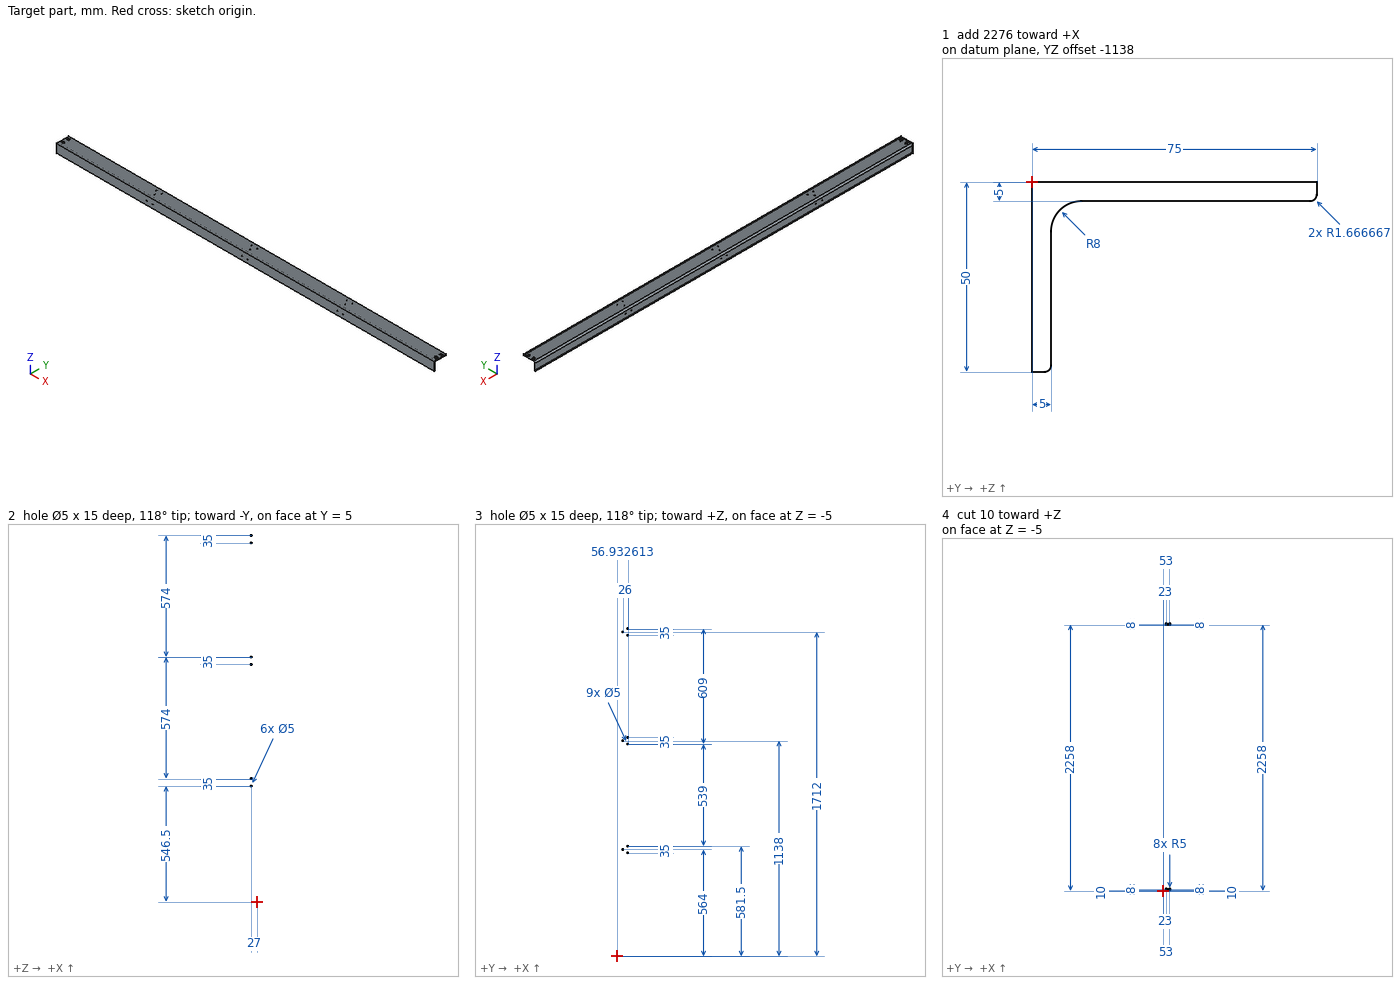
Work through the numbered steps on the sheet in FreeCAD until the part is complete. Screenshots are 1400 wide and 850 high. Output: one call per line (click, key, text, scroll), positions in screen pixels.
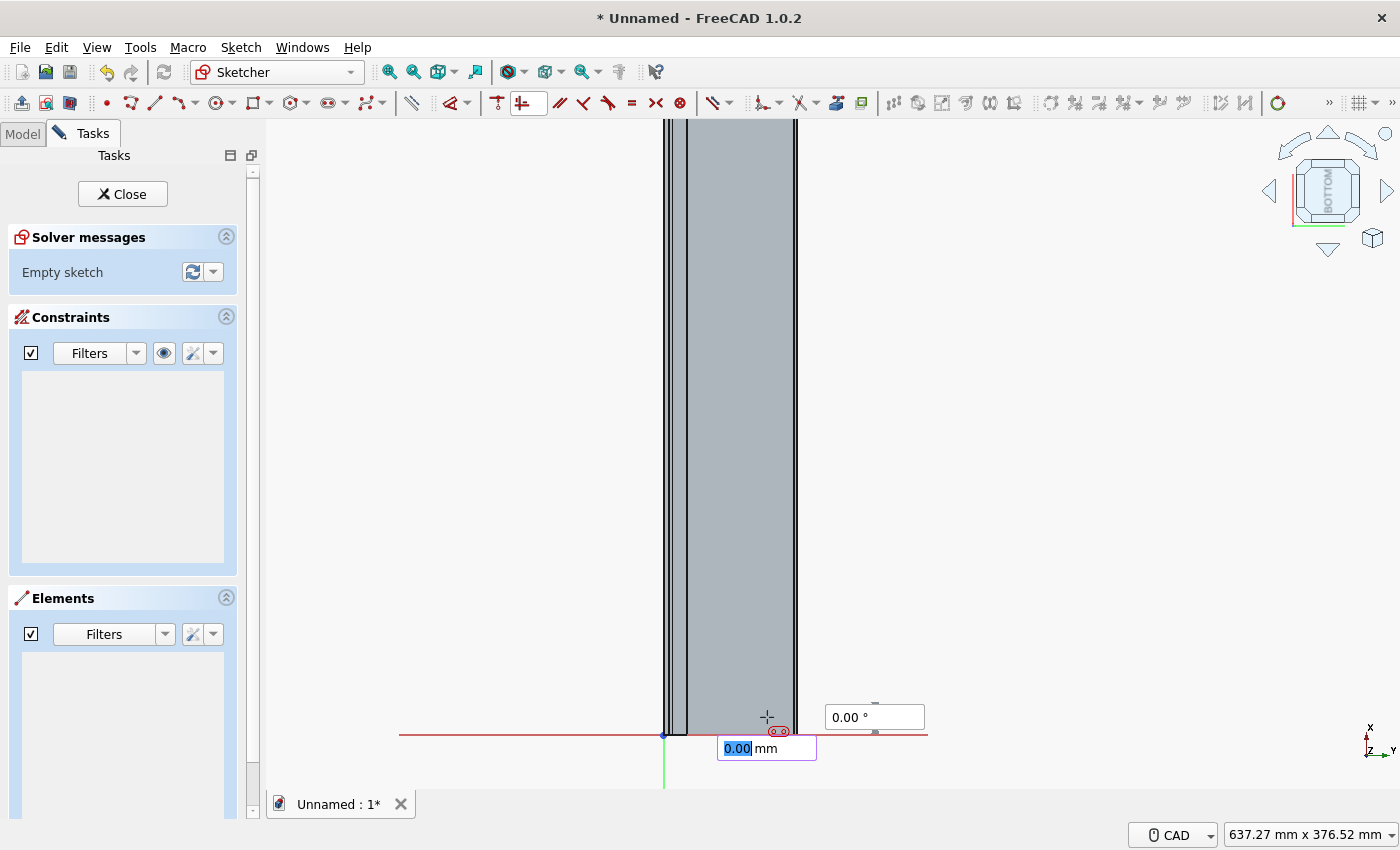
click(767, 703)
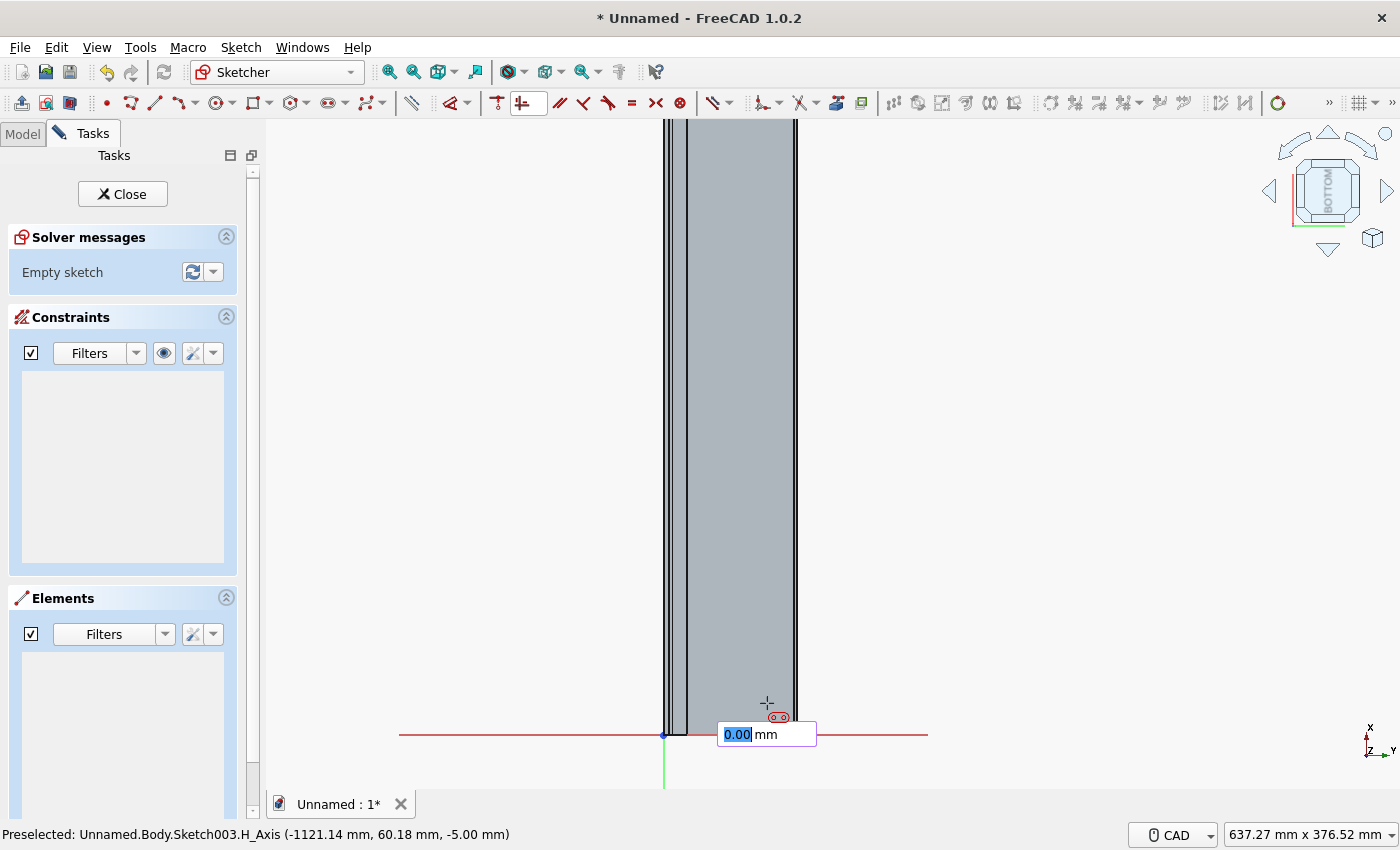
scroll(758, 710, up, 3)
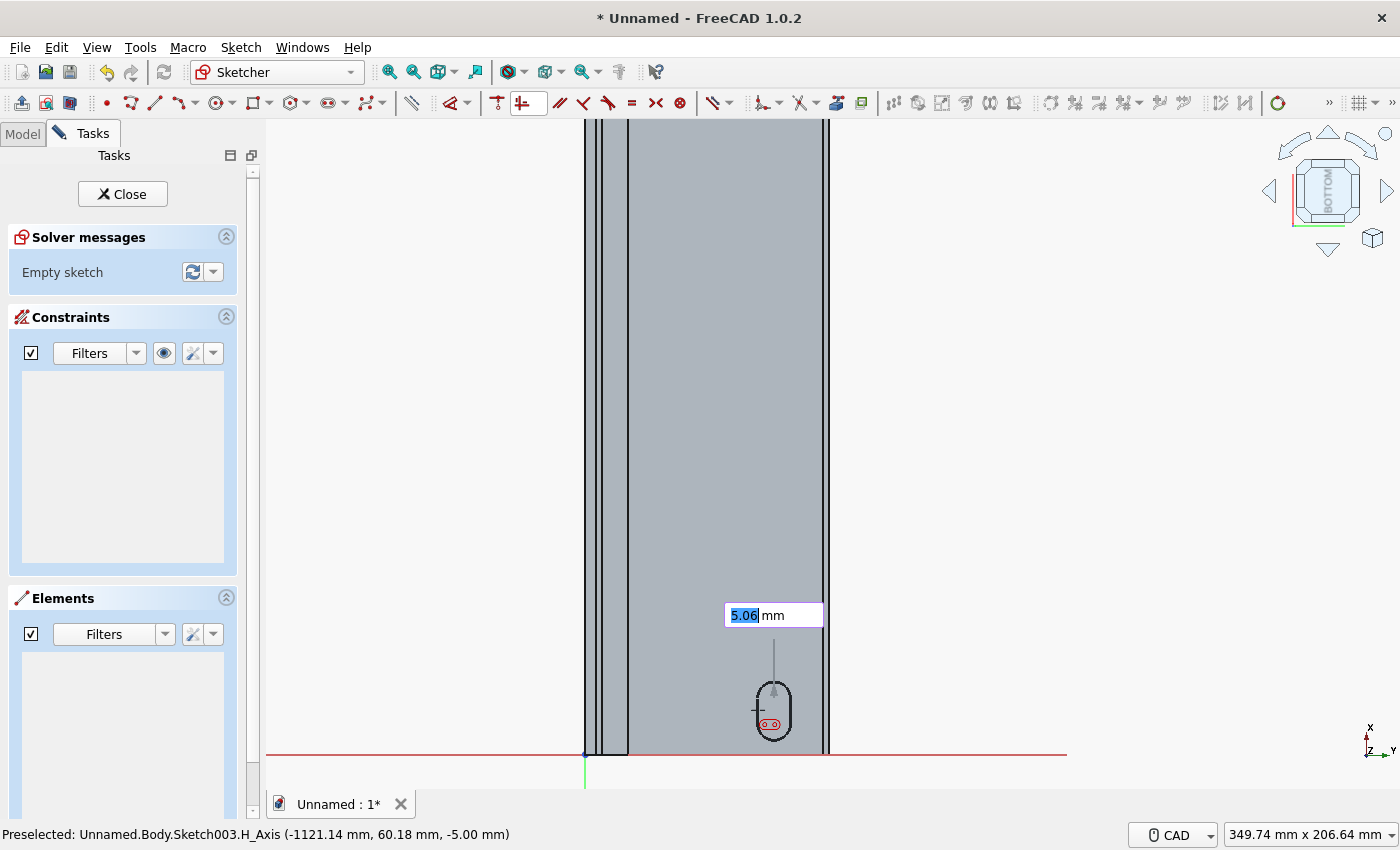
click(757, 709)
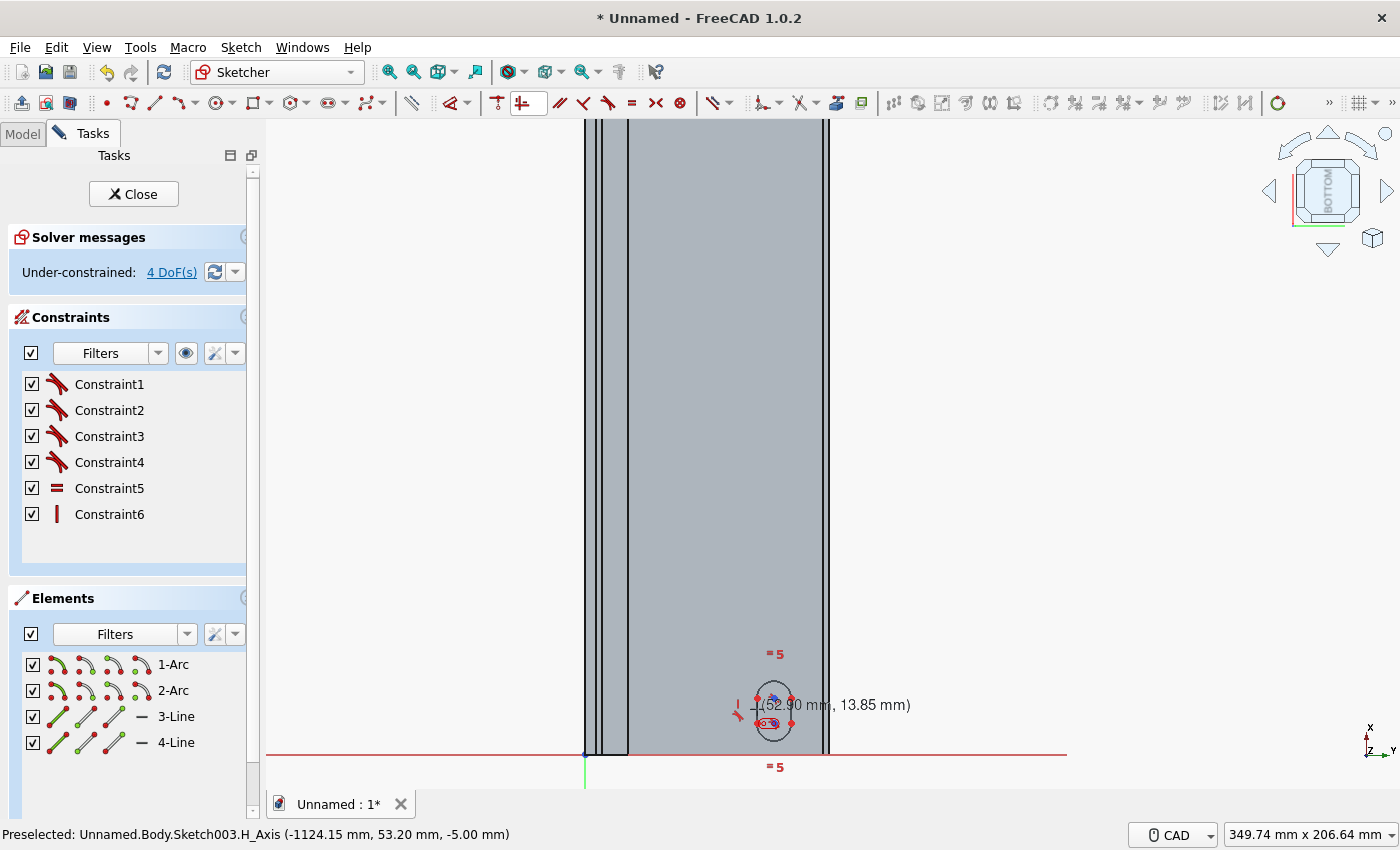
scroll(676, 722, up, 2)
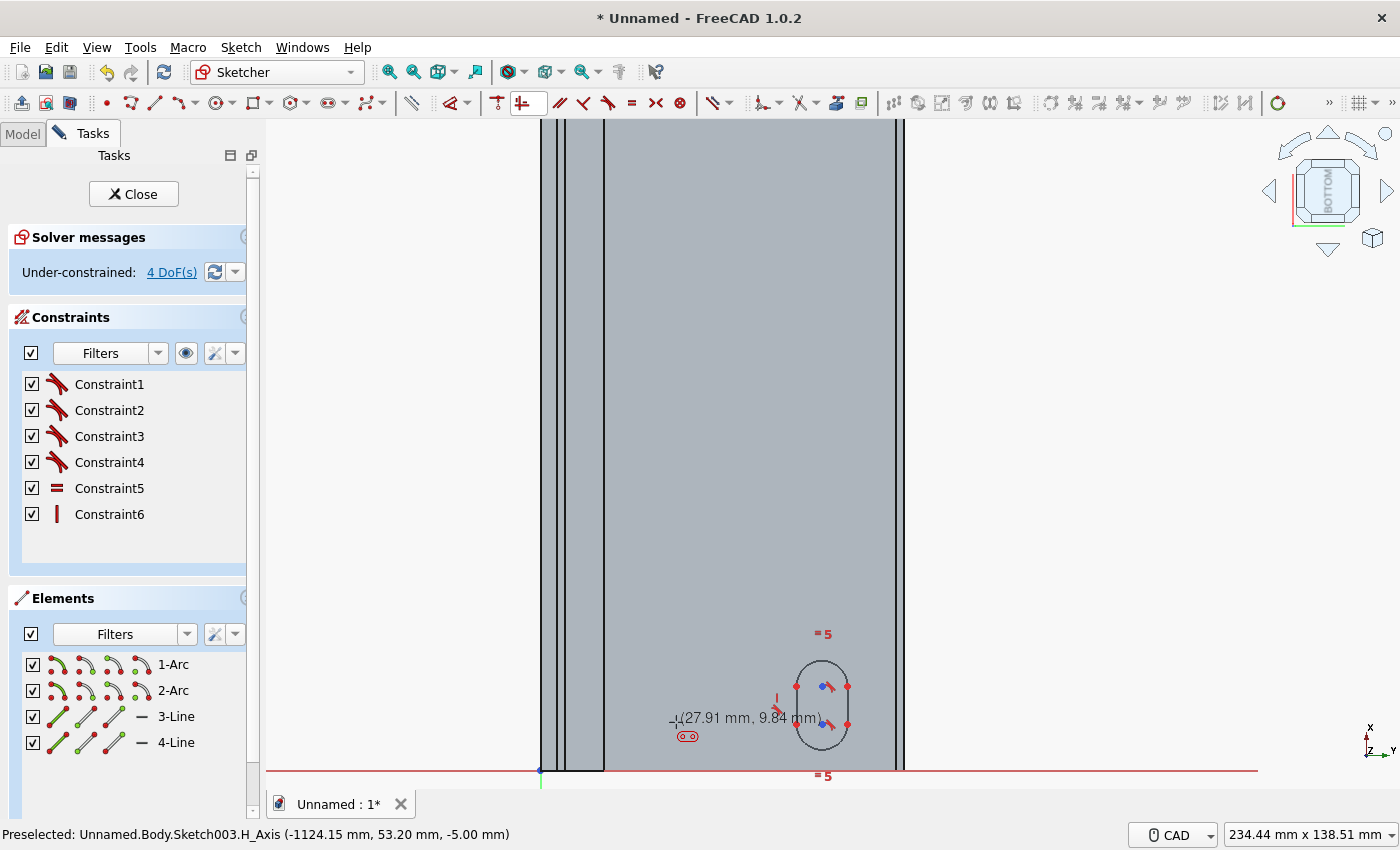
scroll(768, 725, down, 15)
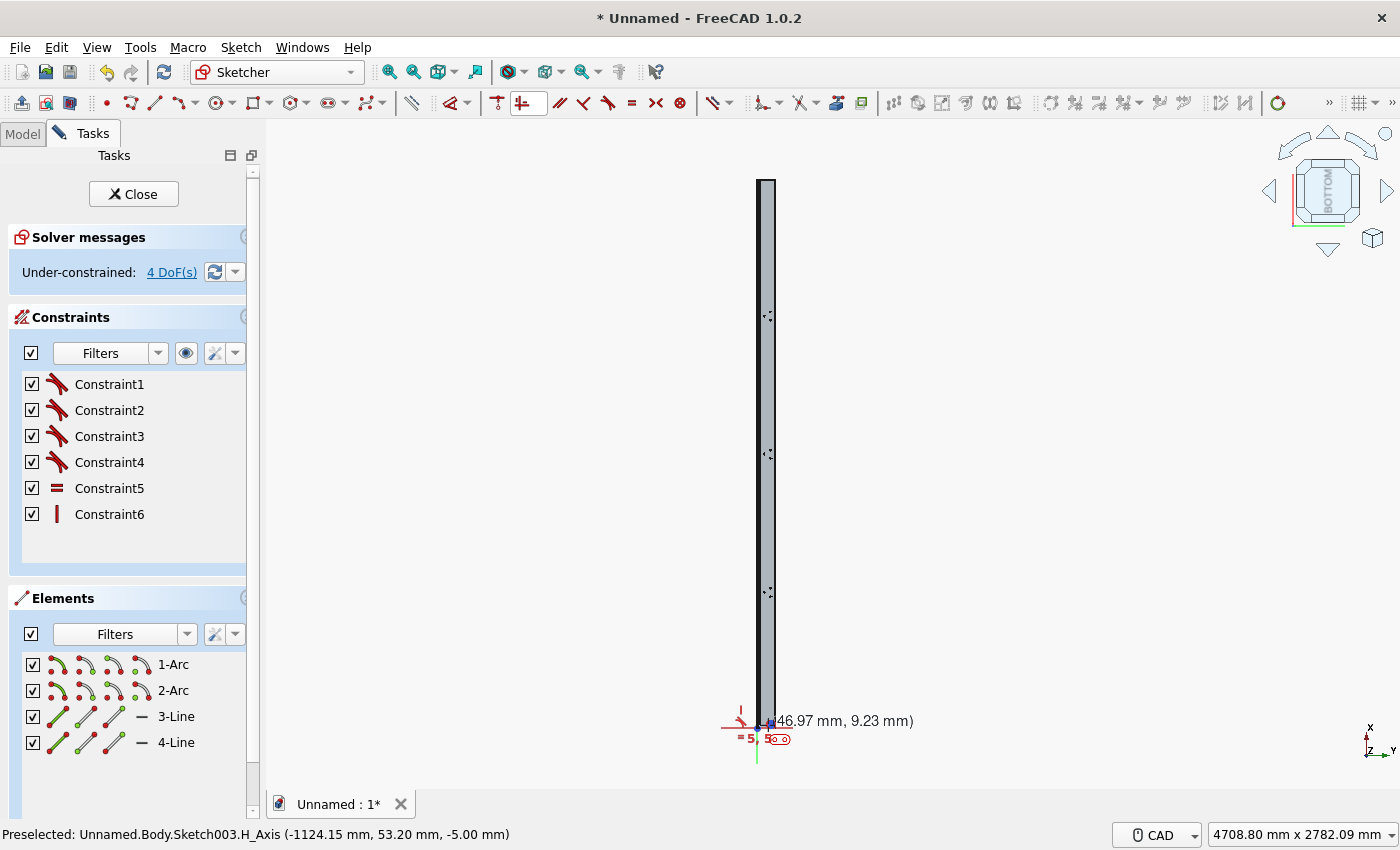
scroll(764, 726, up, 10)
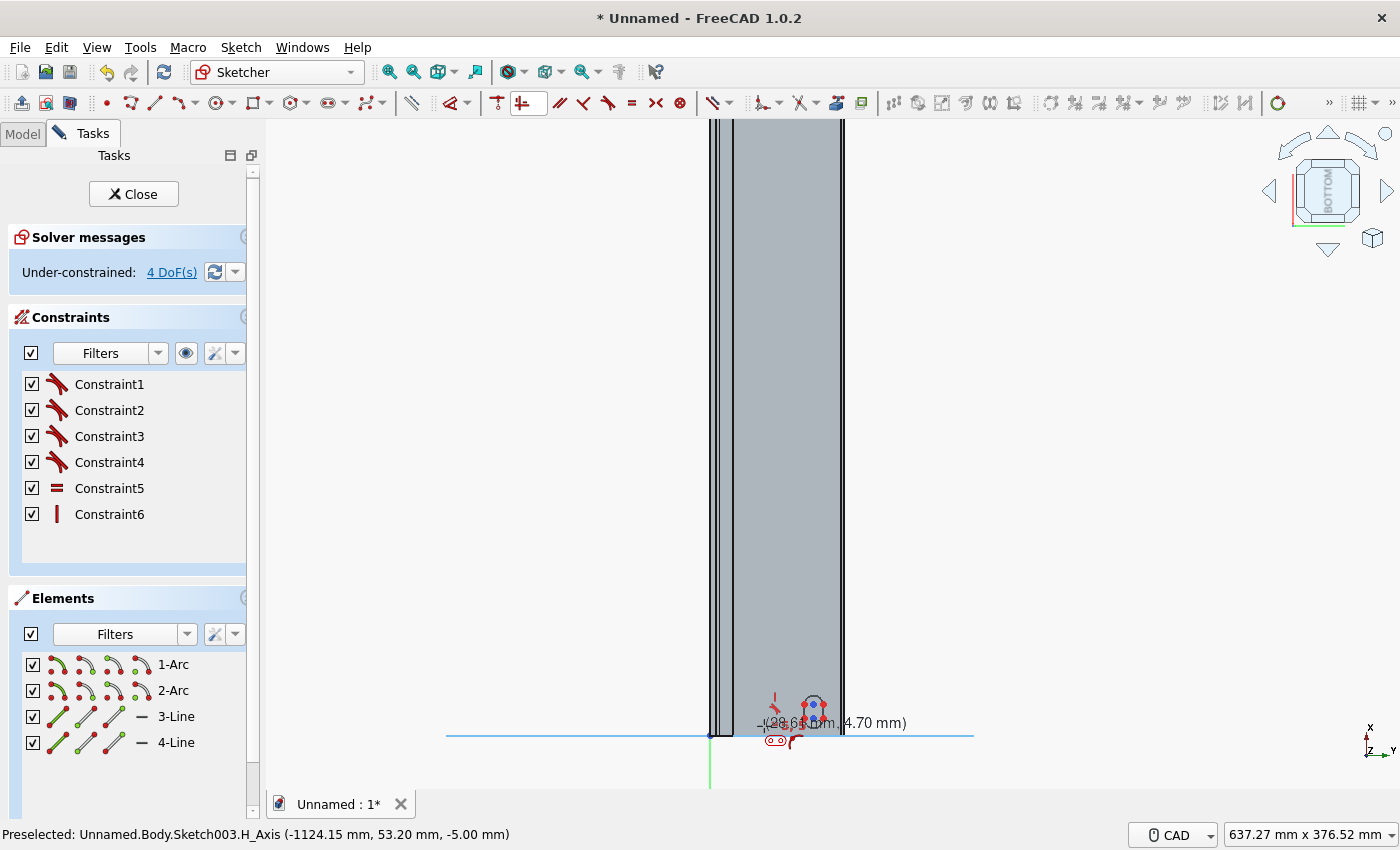
click(760, 718)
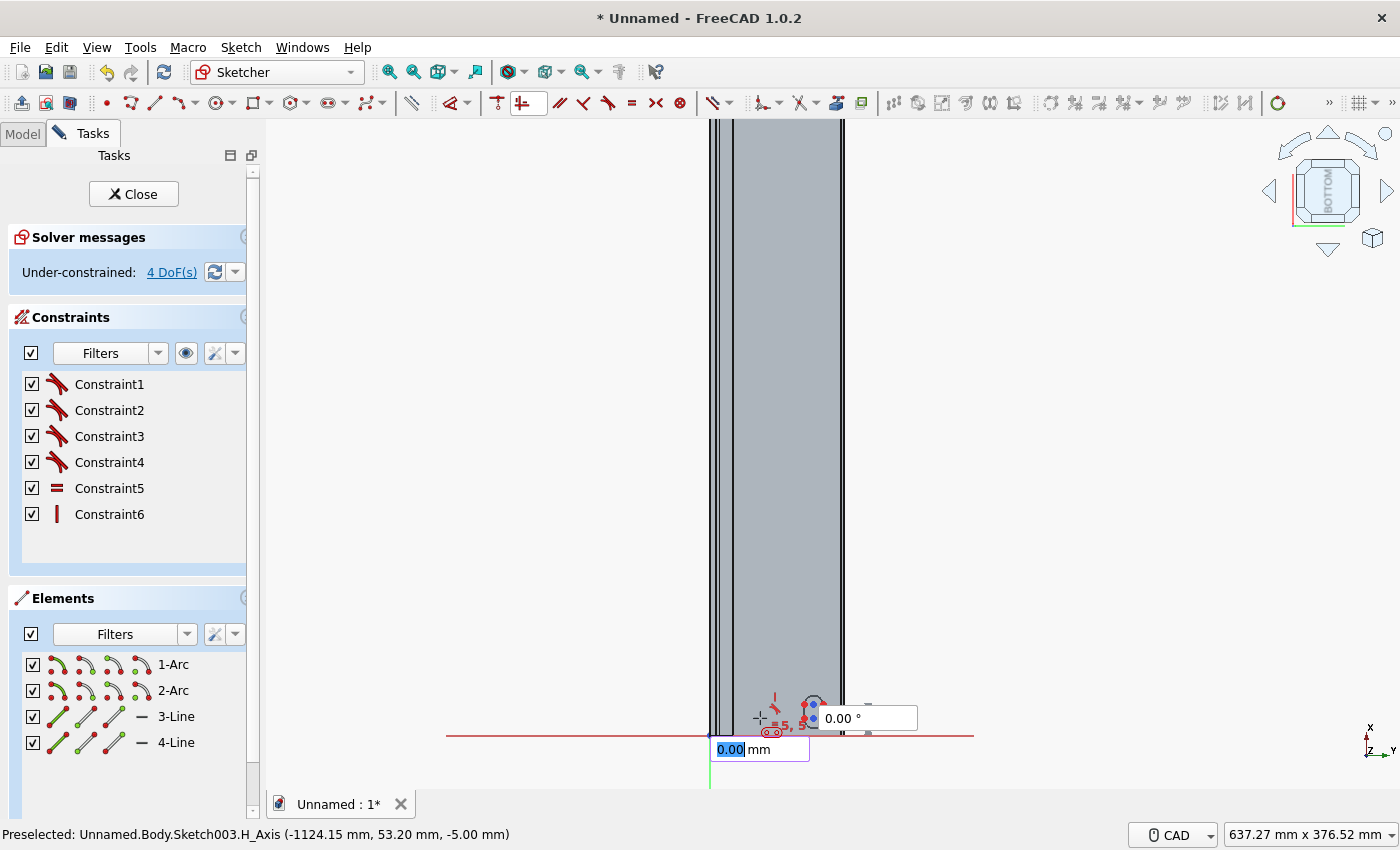
click(760, 704)